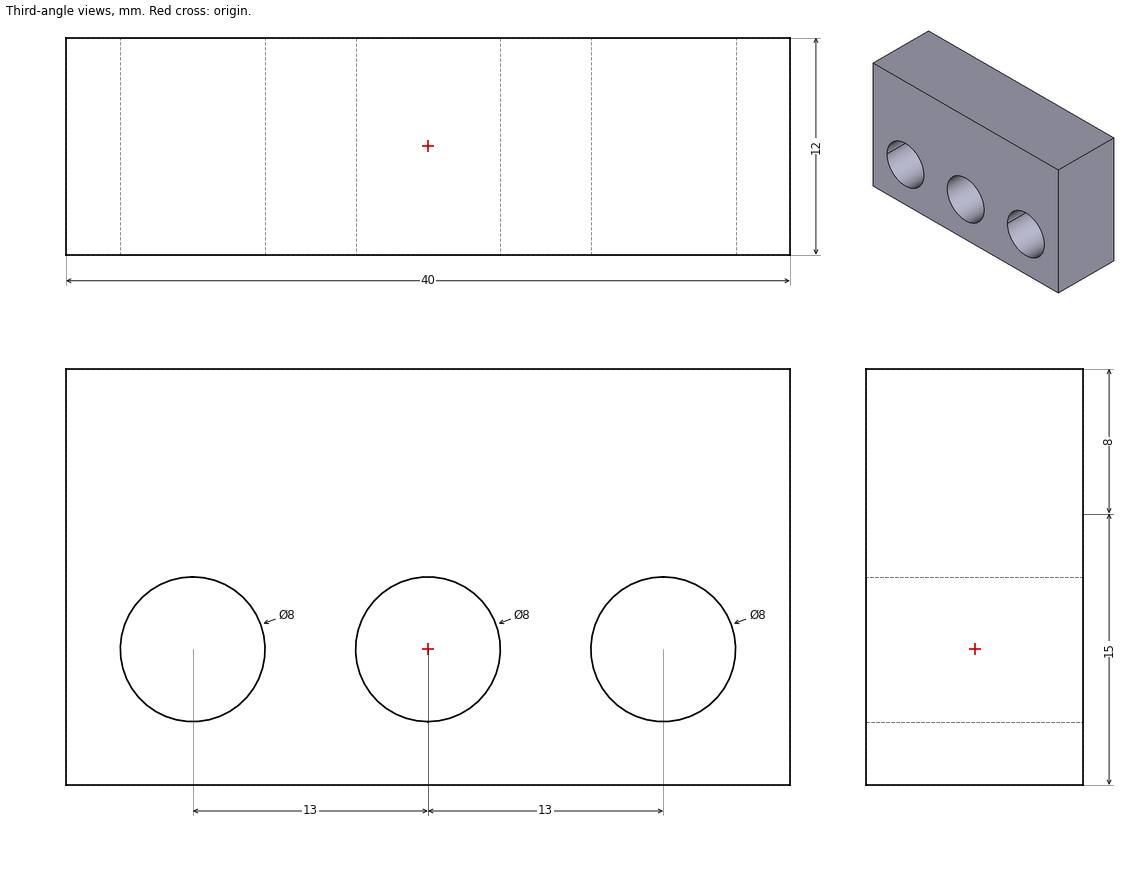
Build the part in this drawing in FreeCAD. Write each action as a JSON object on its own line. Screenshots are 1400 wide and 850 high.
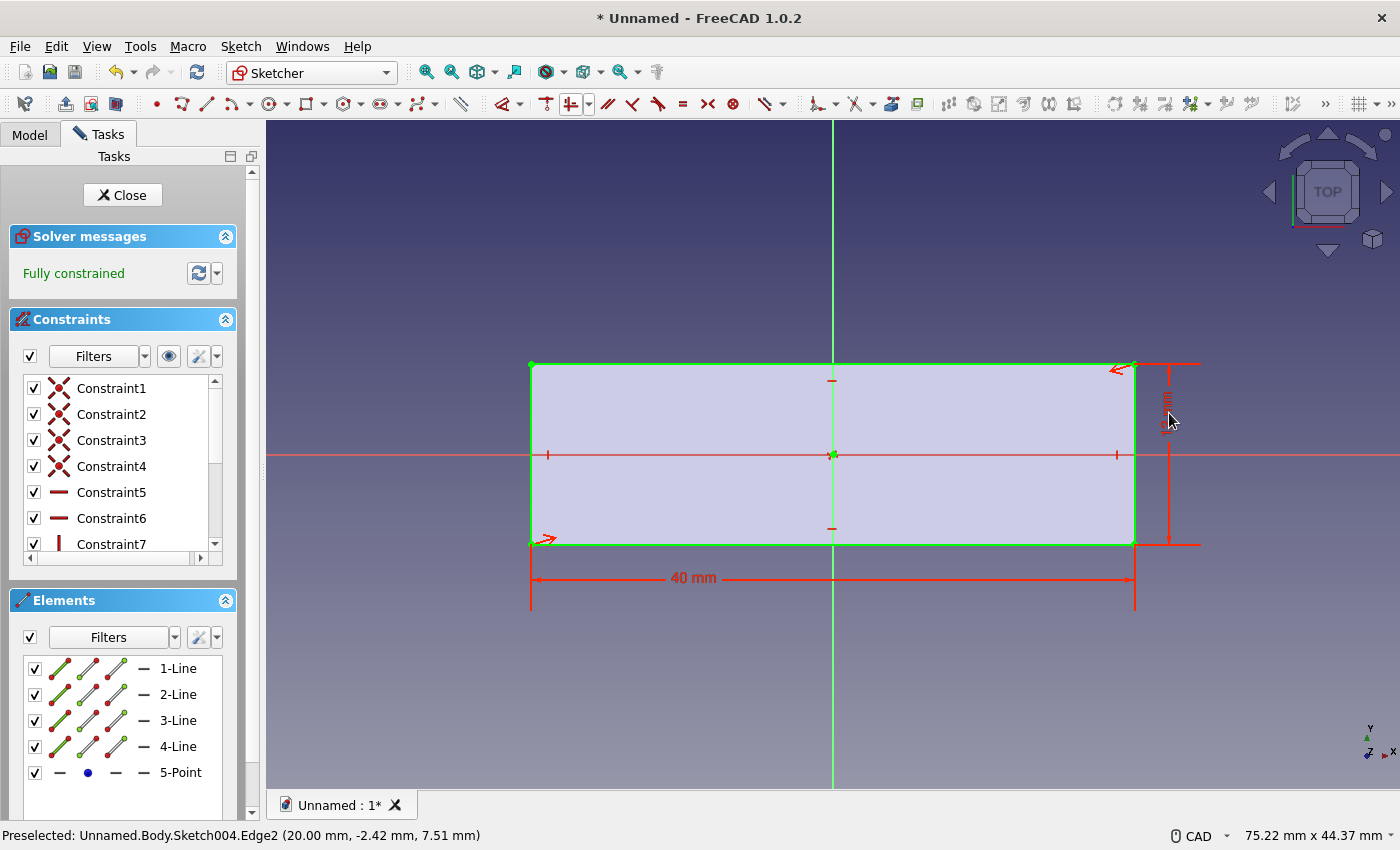
{"action": "left_click", "coordinate": [123, 195]}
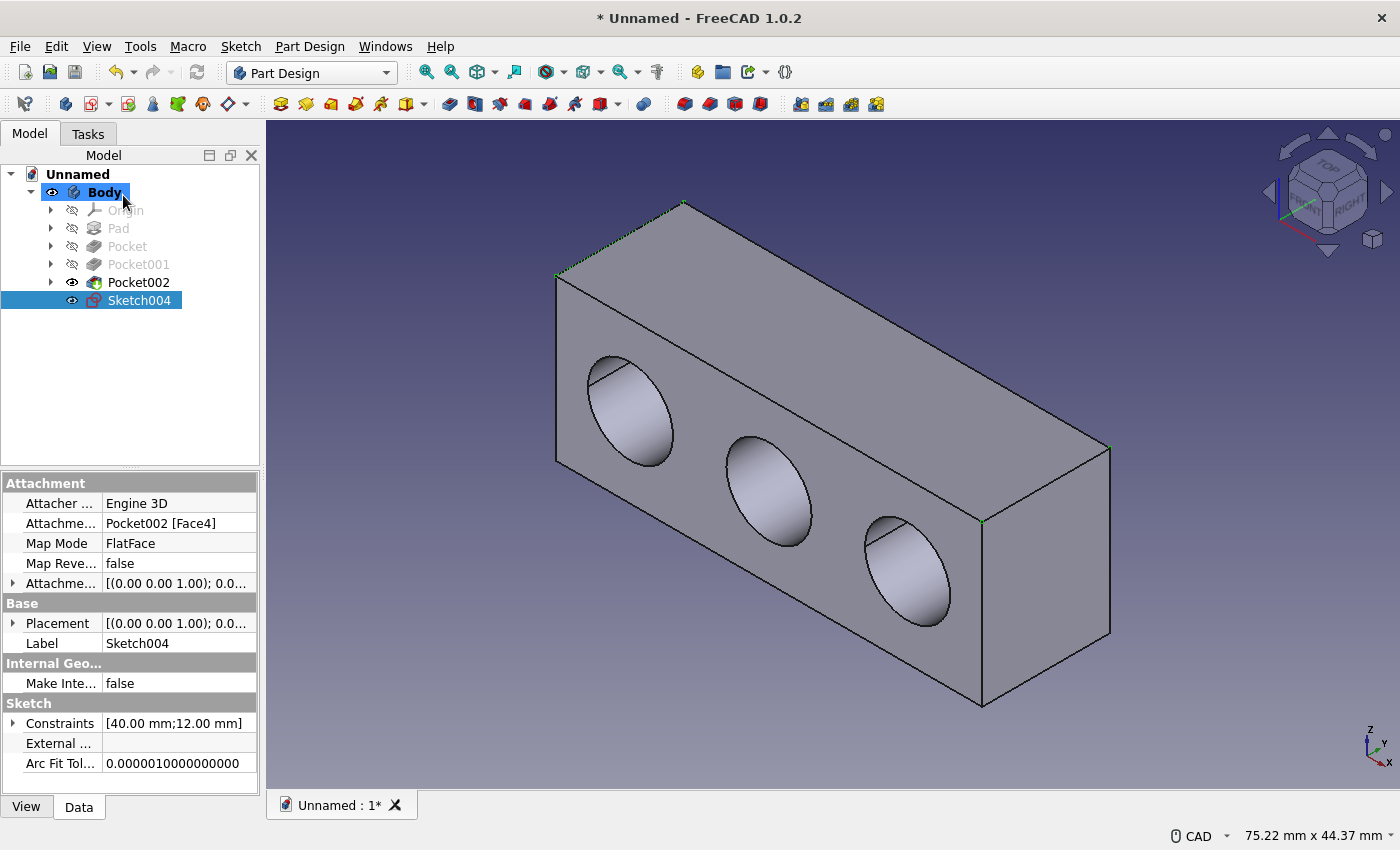
{"action": "left_click", "coordinate": [281, 104]}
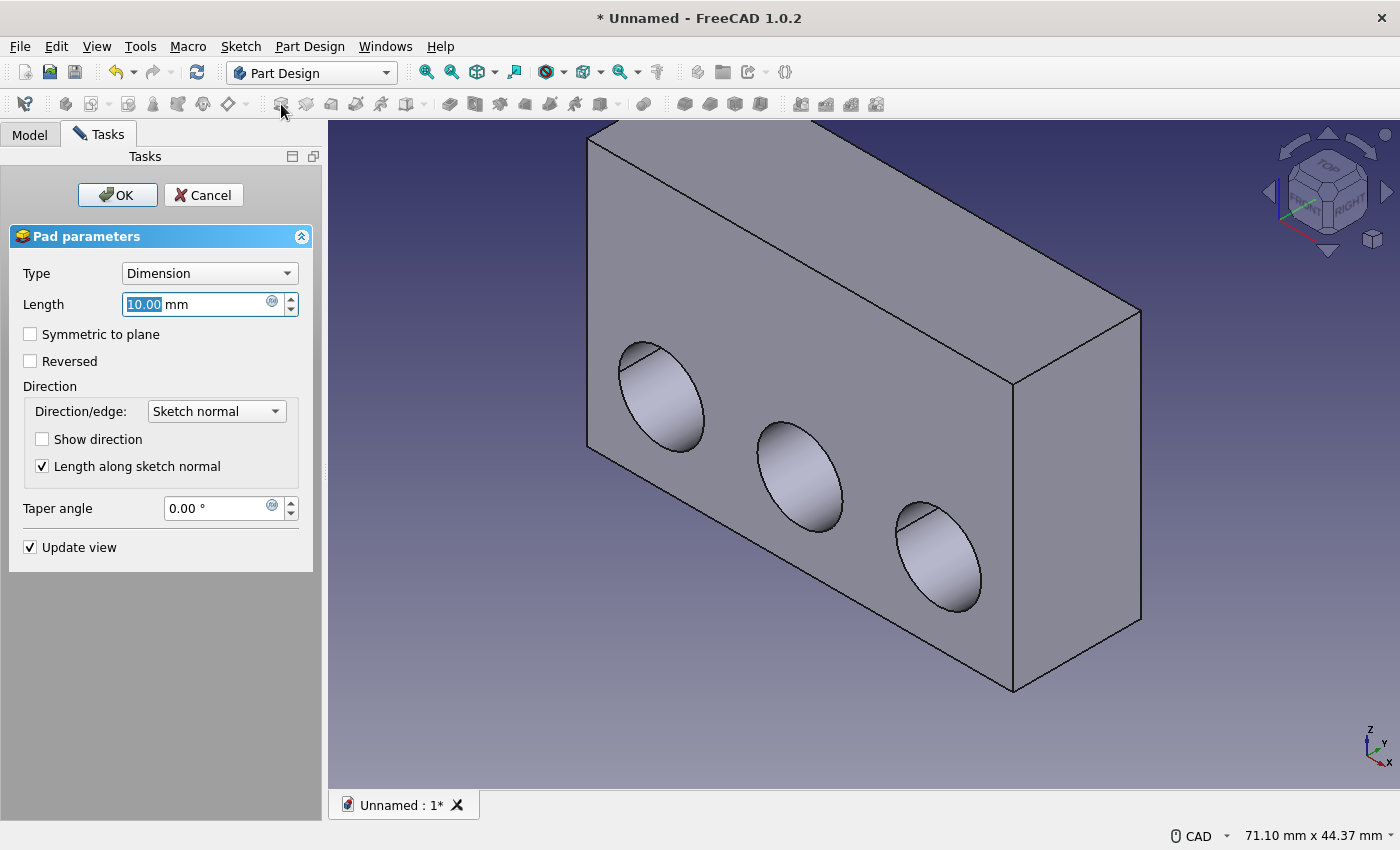
{"action": "type", "text": "8"}
{"action": "key", "text": "Tab"}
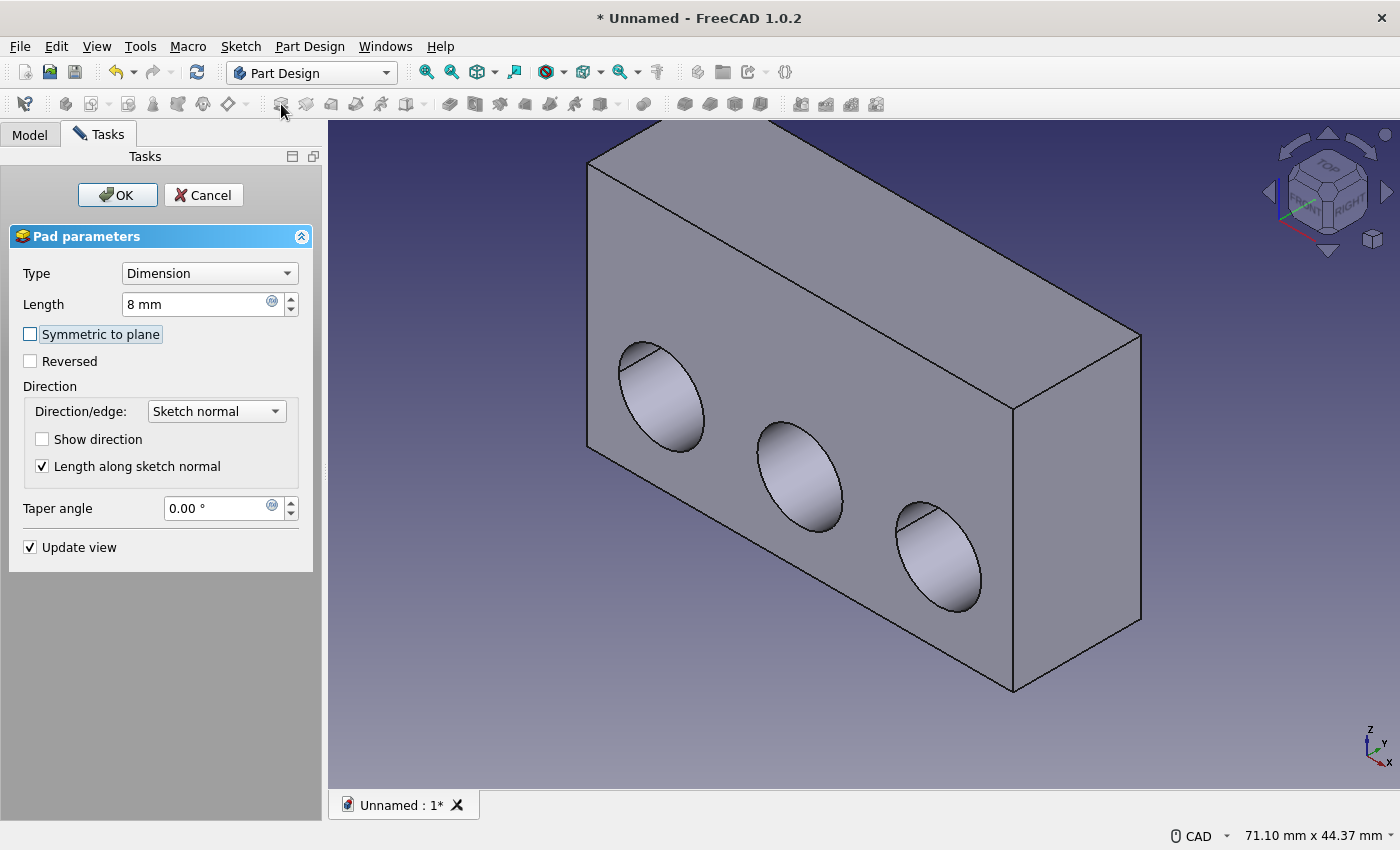
{"action": "left_click", "coordinate": [118, 195]}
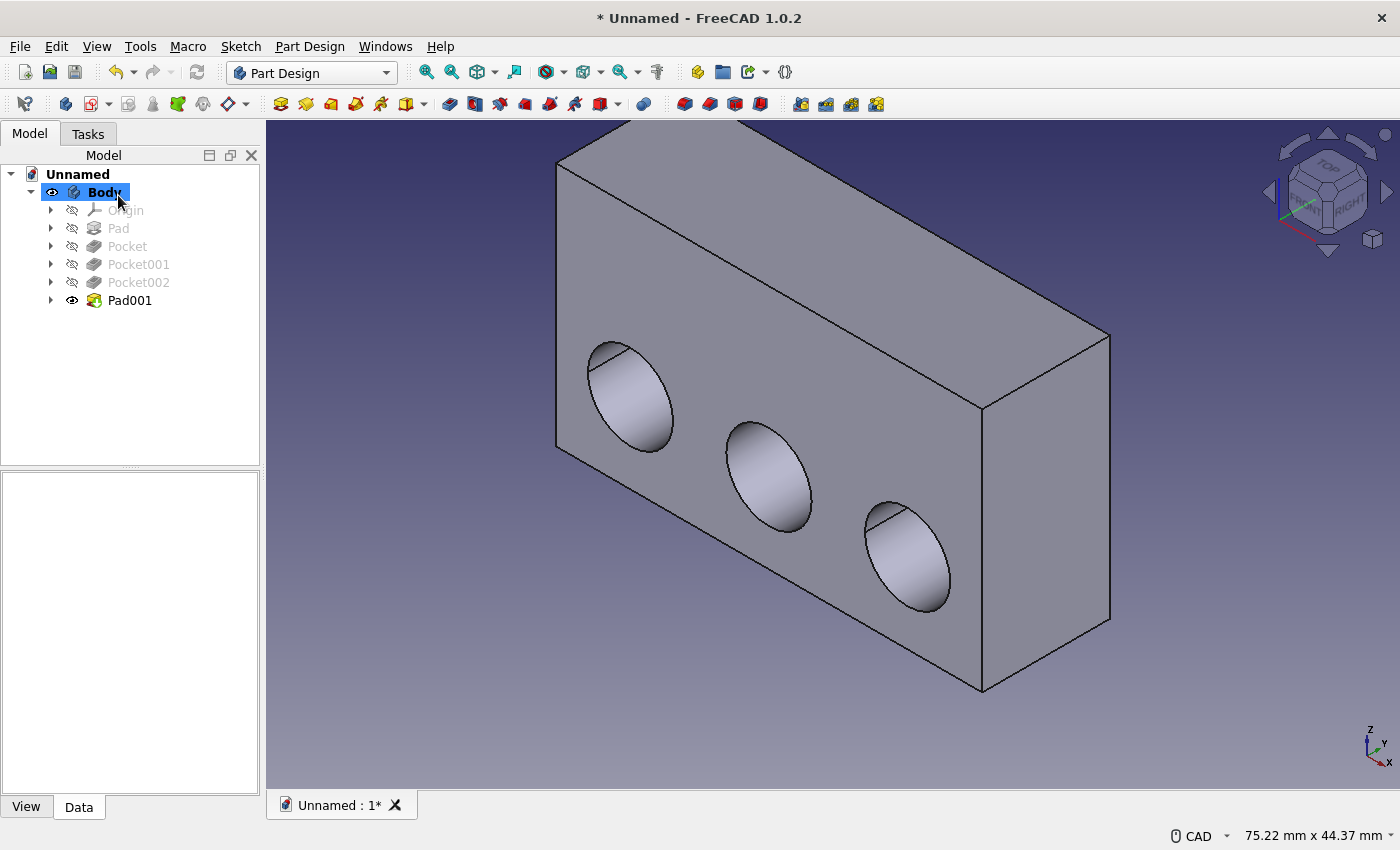
{"action": "key", "text": "v f"}